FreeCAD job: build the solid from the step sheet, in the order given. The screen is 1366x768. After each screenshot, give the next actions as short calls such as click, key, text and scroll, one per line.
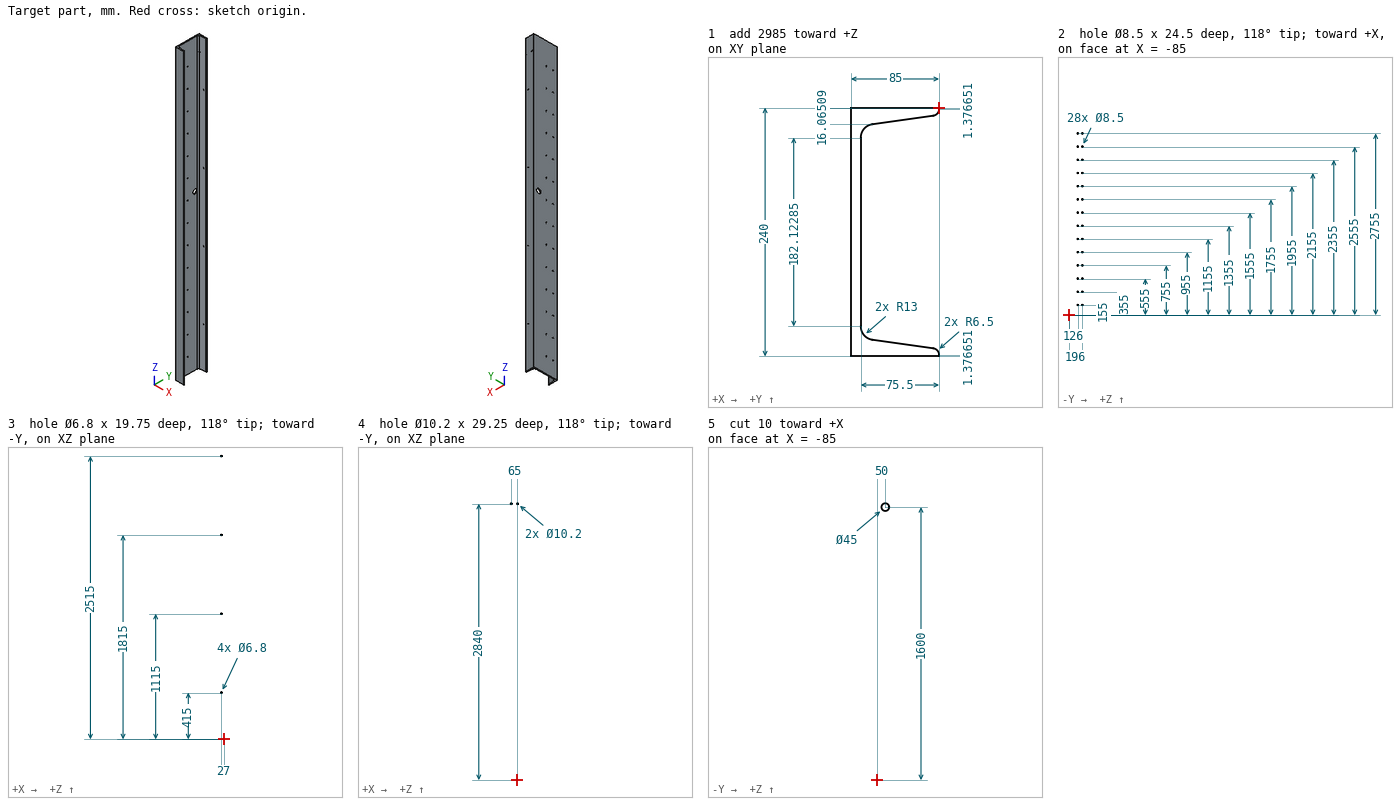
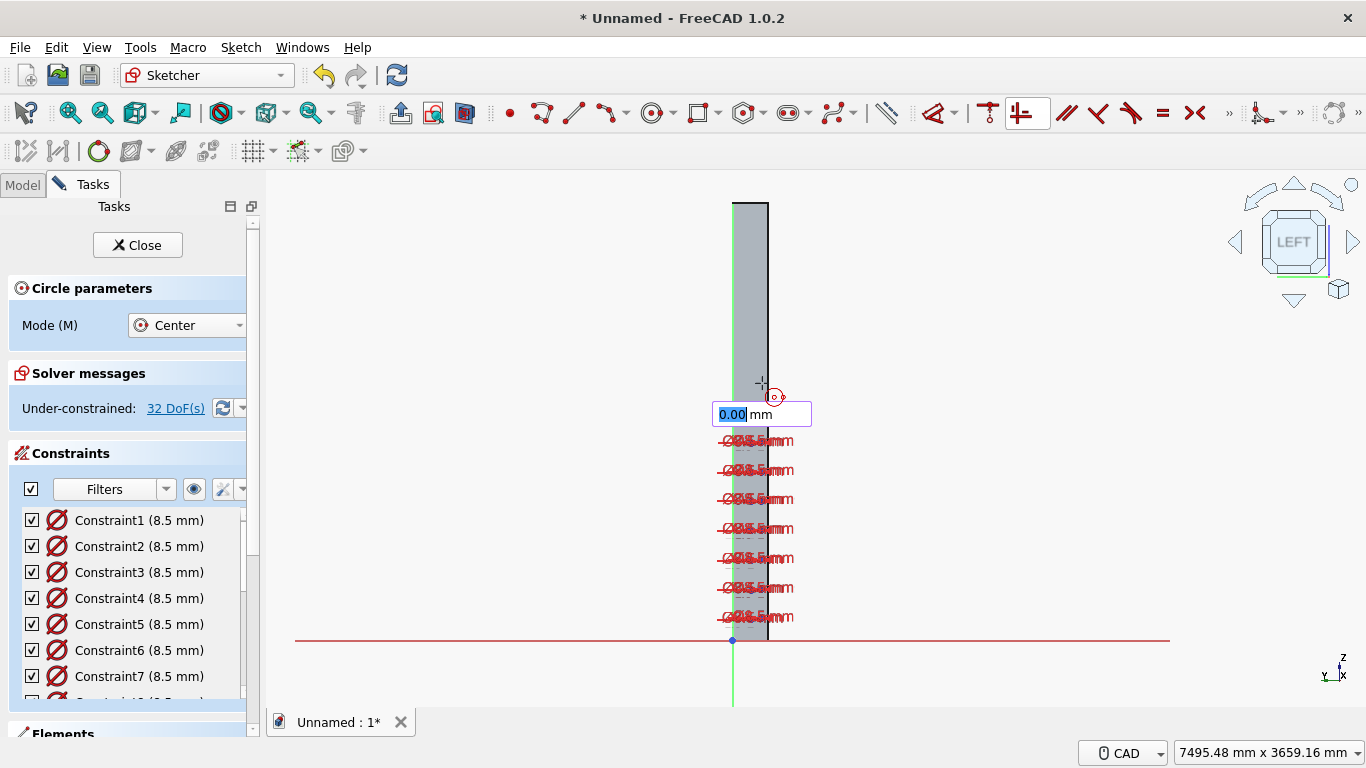
text(8.5)
key(Return)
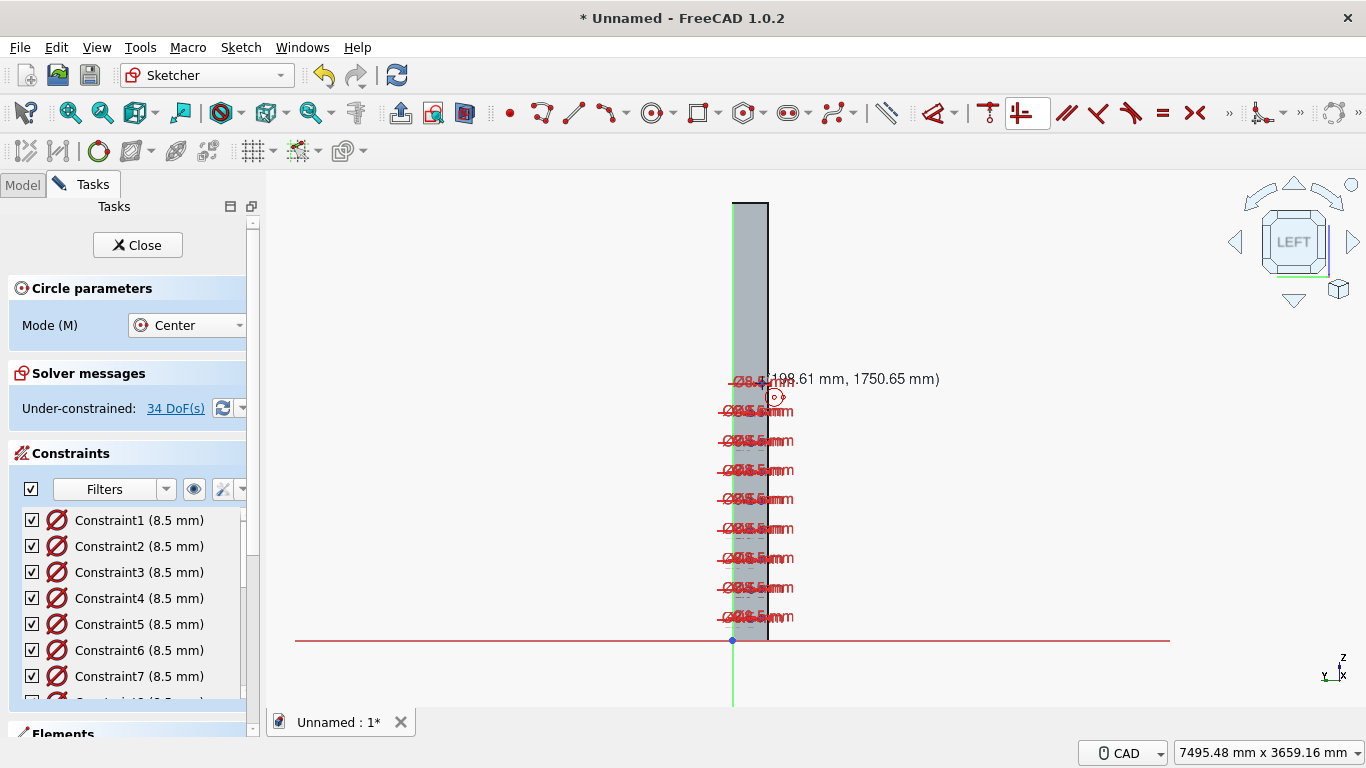
scroll(751, 383, up, 18)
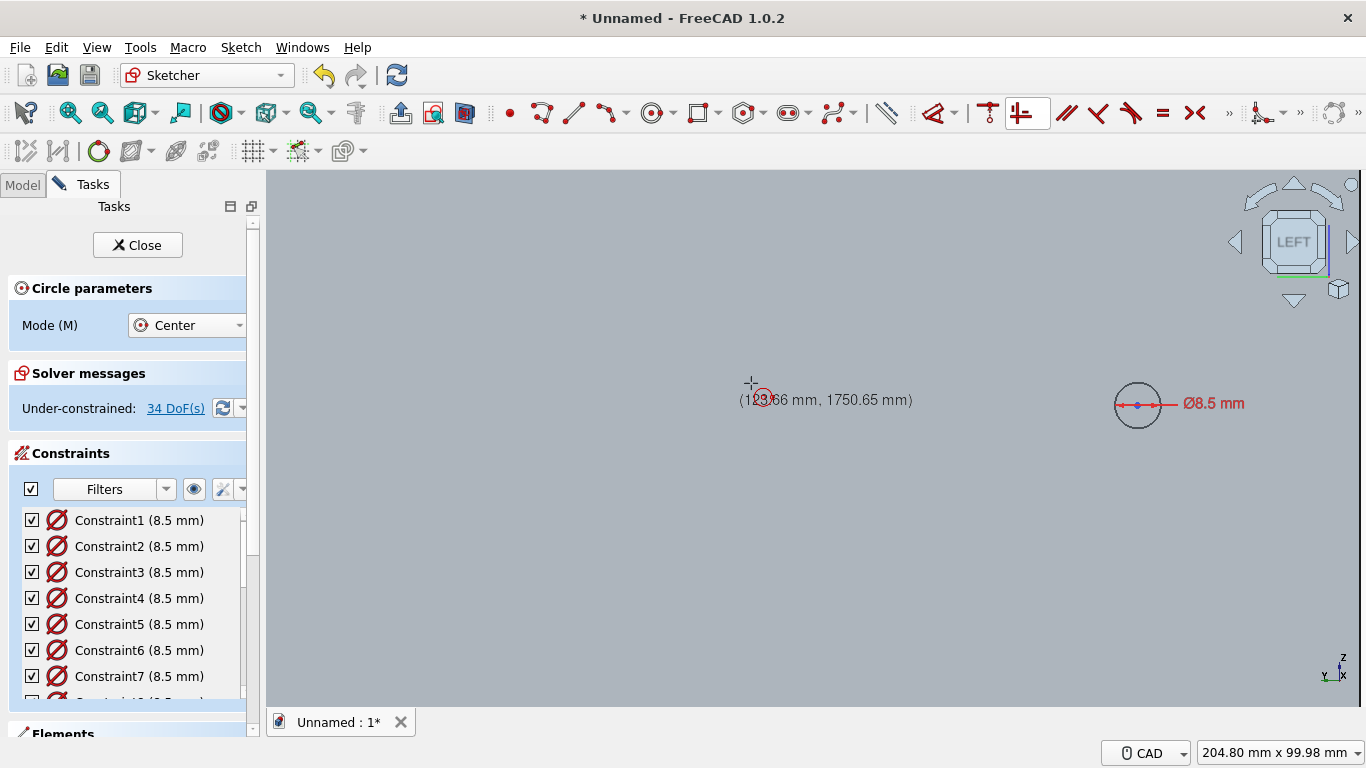
scroll(751, 383, down, 18)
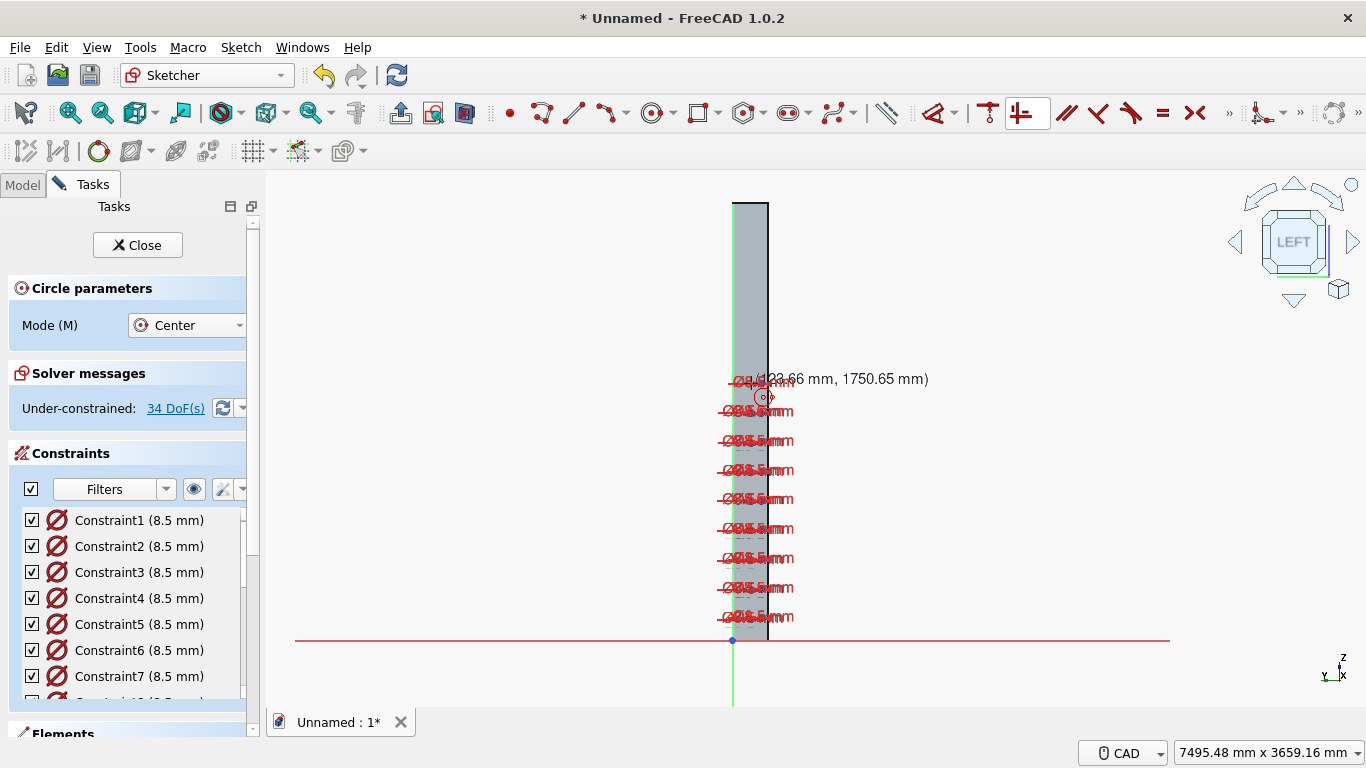
scroll(751, 383, up, 3)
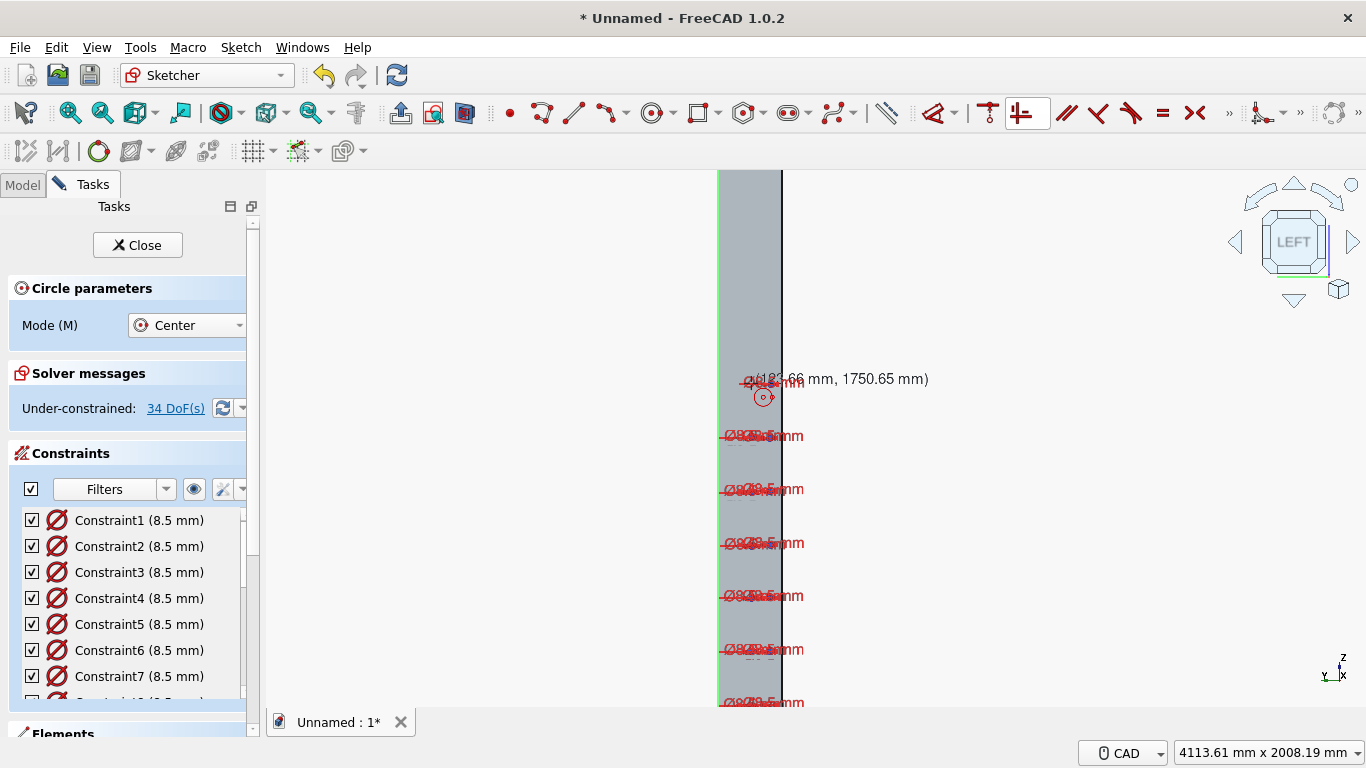
click(751, 383)
move(752, 383)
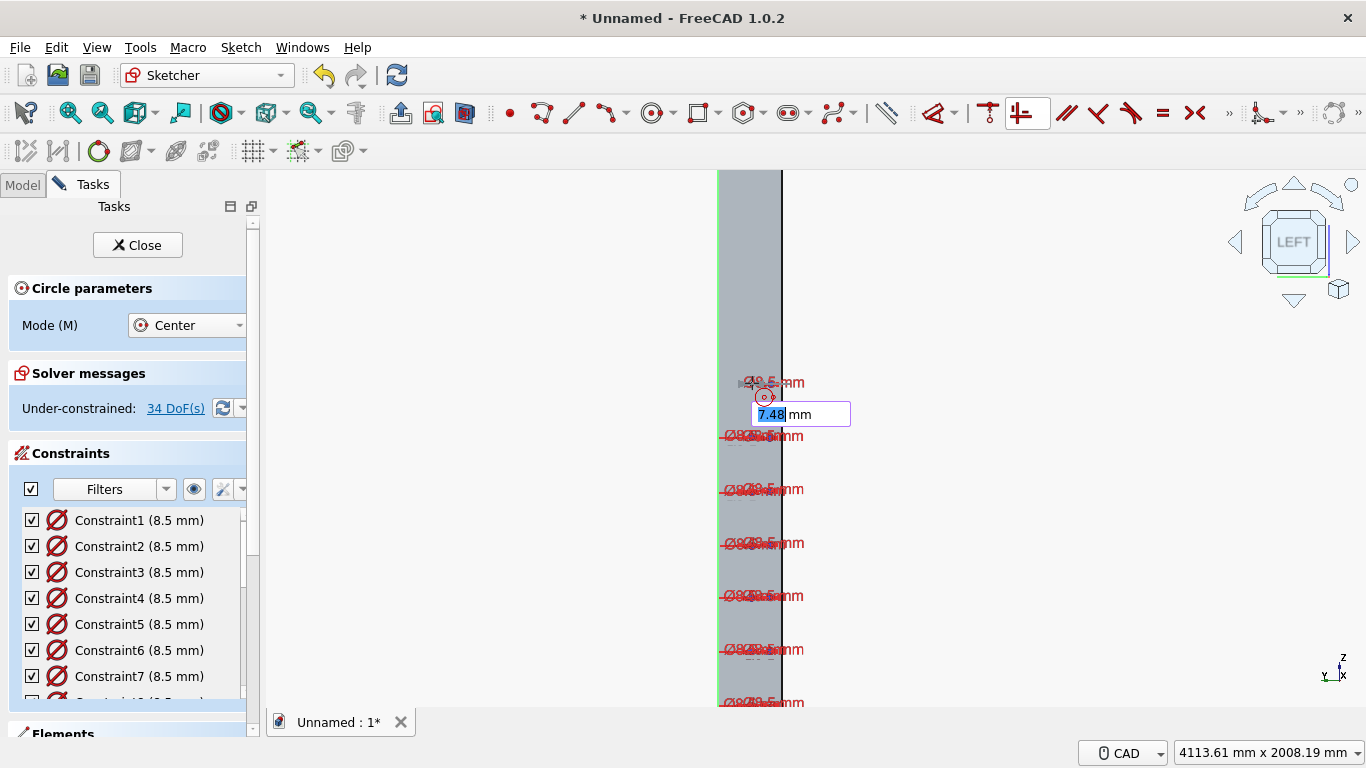
text(8.5)
key(Return)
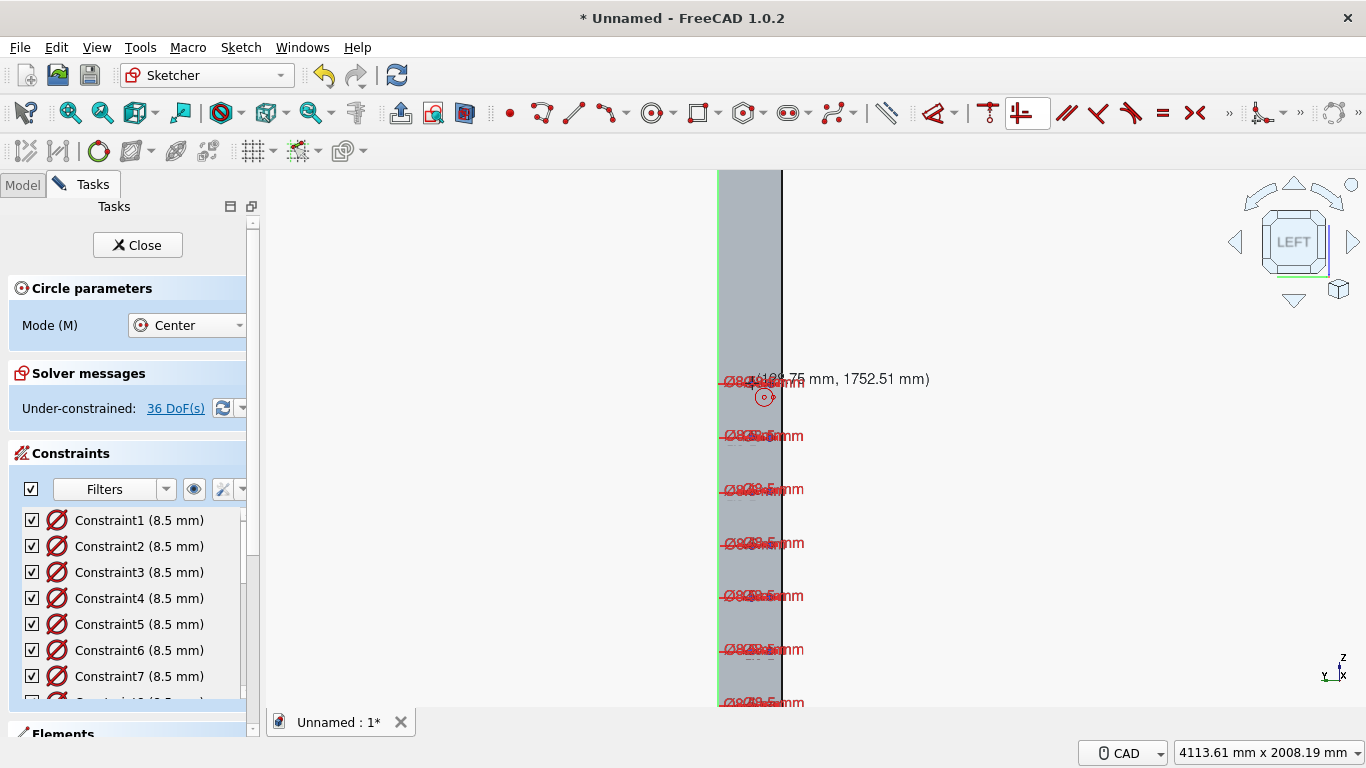
scroll(751, 330, up, 15)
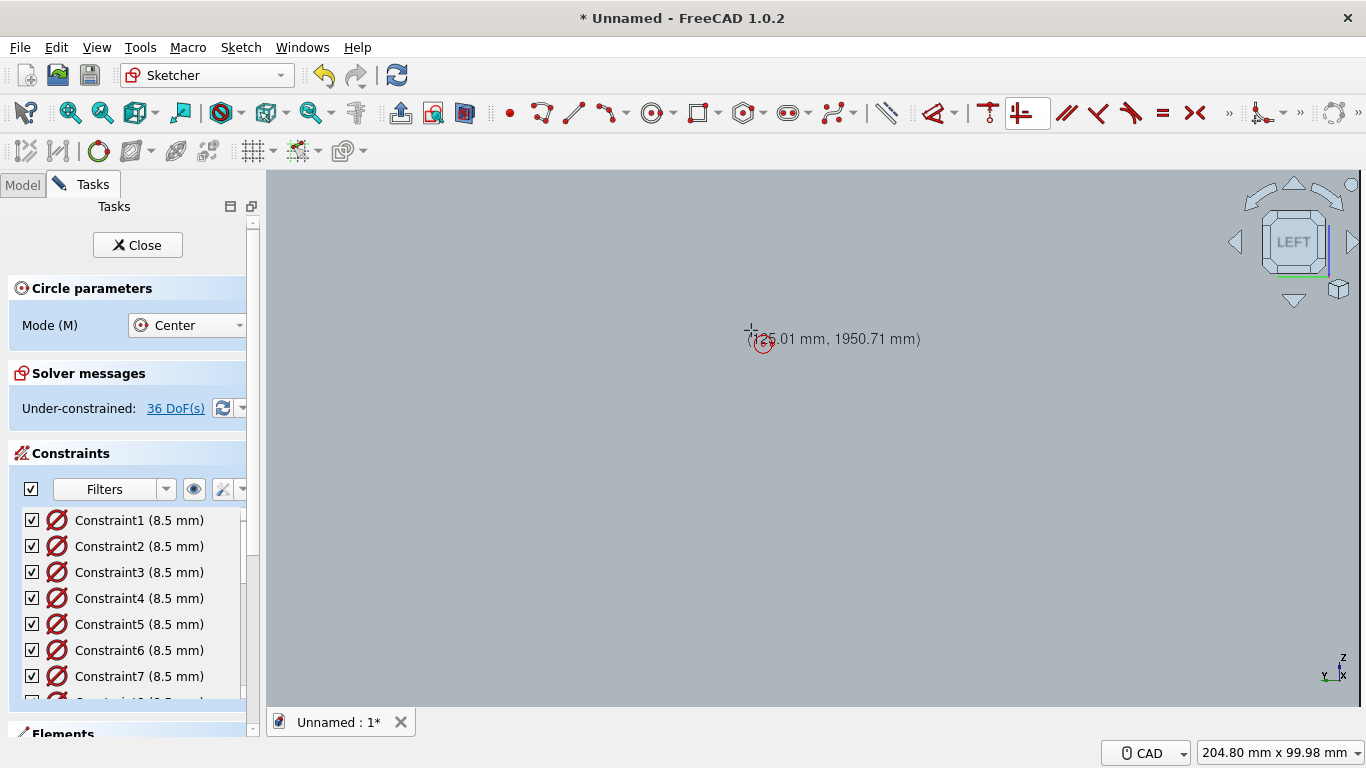
scroll(751, 355, down, 18)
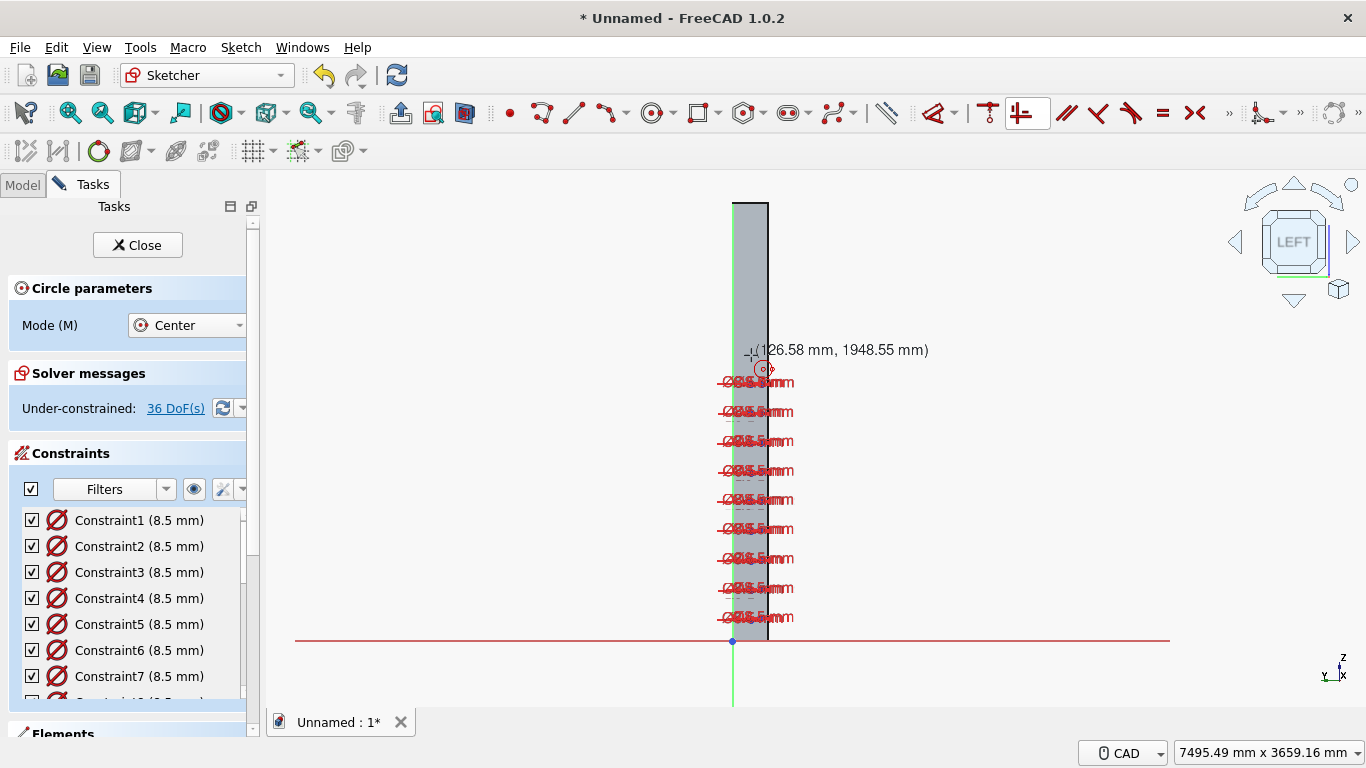
click(751, 354)
move(752, 354)